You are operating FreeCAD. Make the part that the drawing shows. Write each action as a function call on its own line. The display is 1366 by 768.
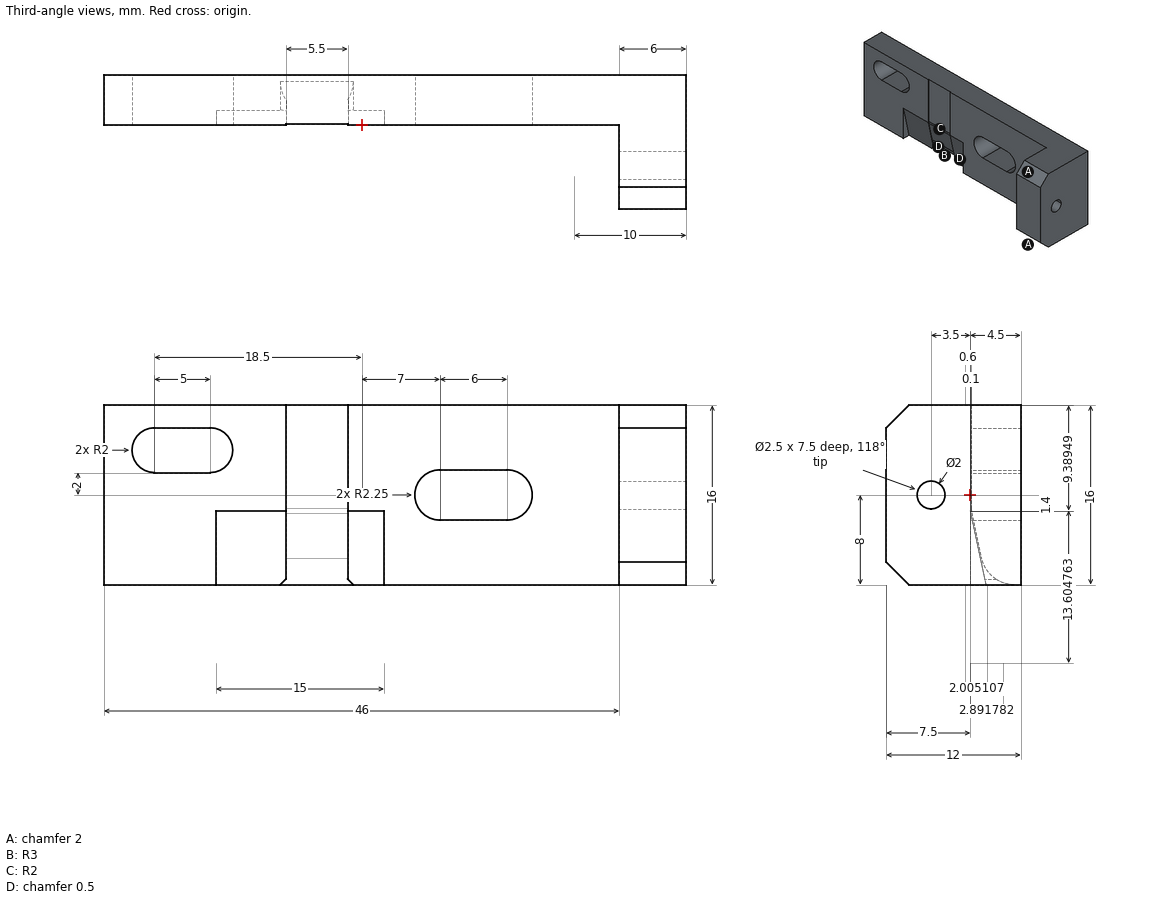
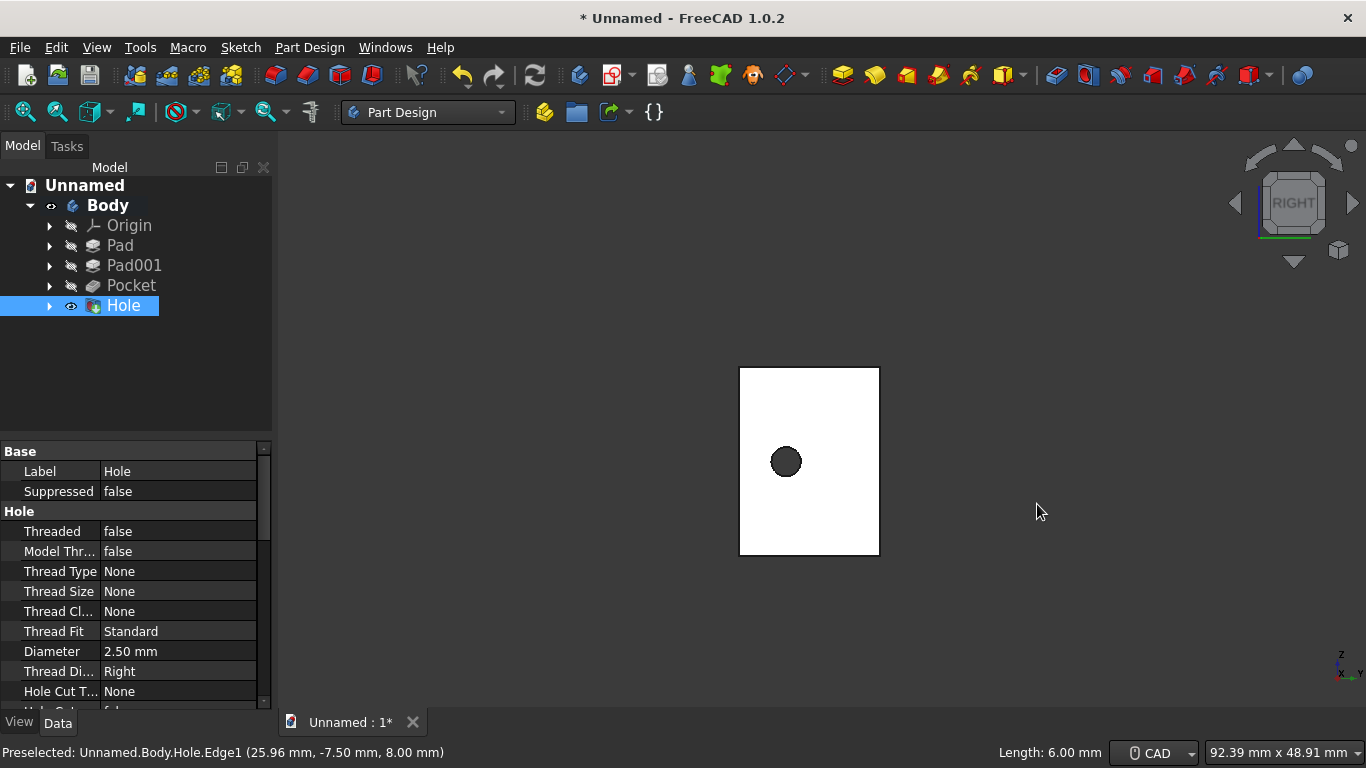
key(v)
key(f)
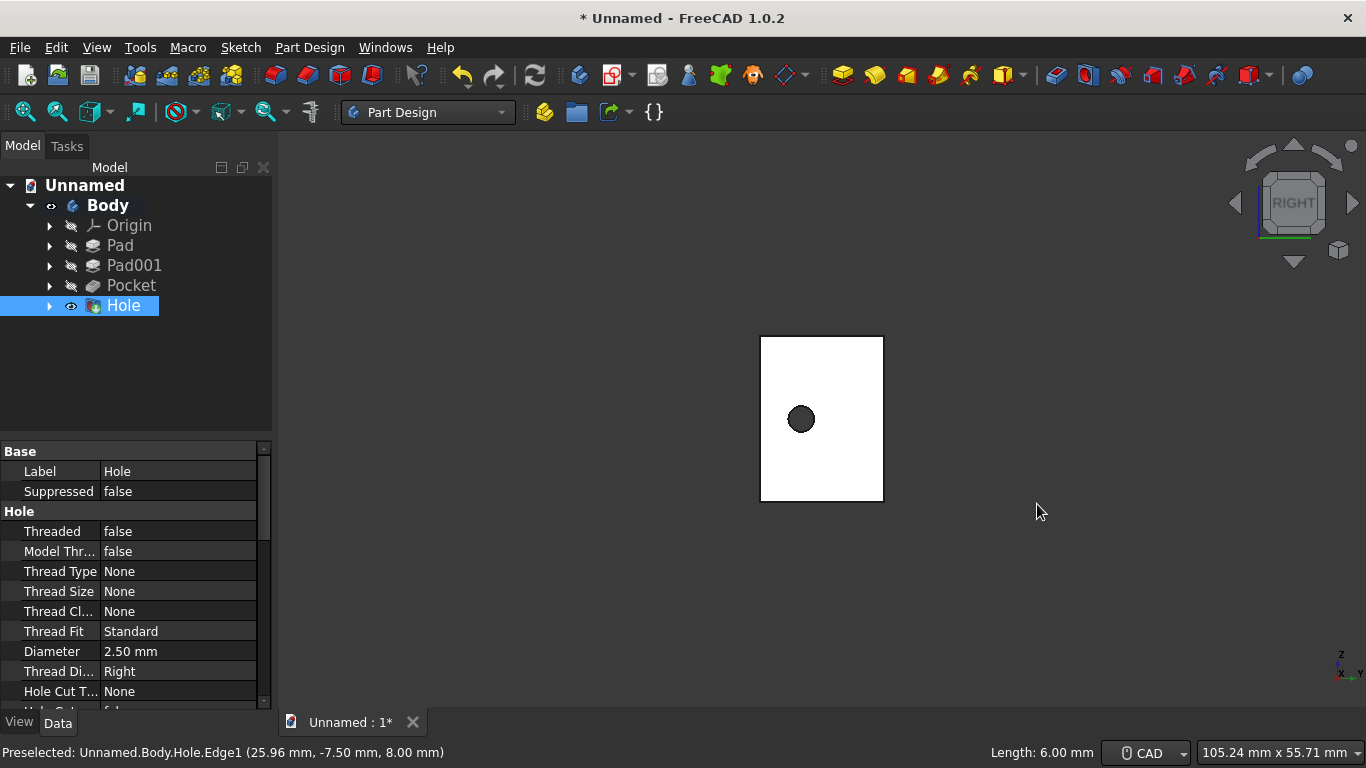
key(5)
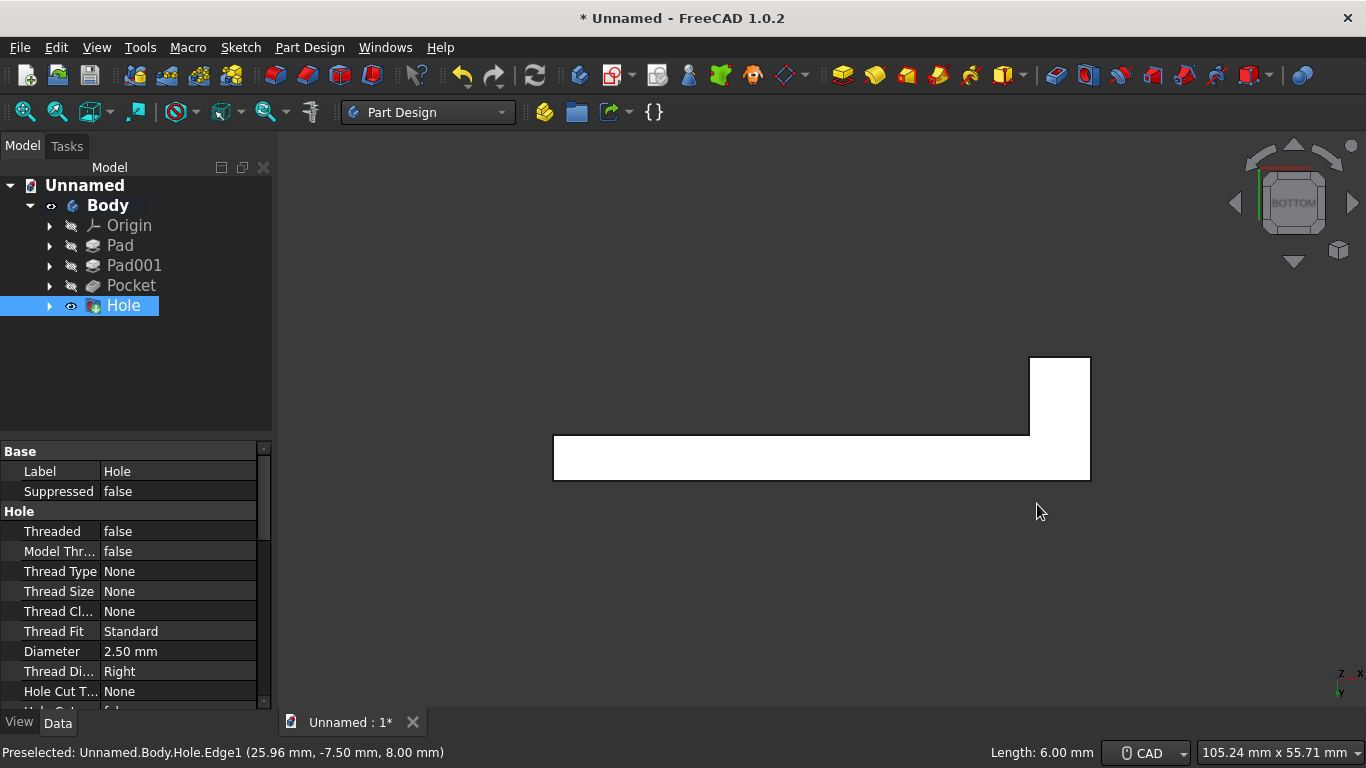
click(1060, 356, ctrl)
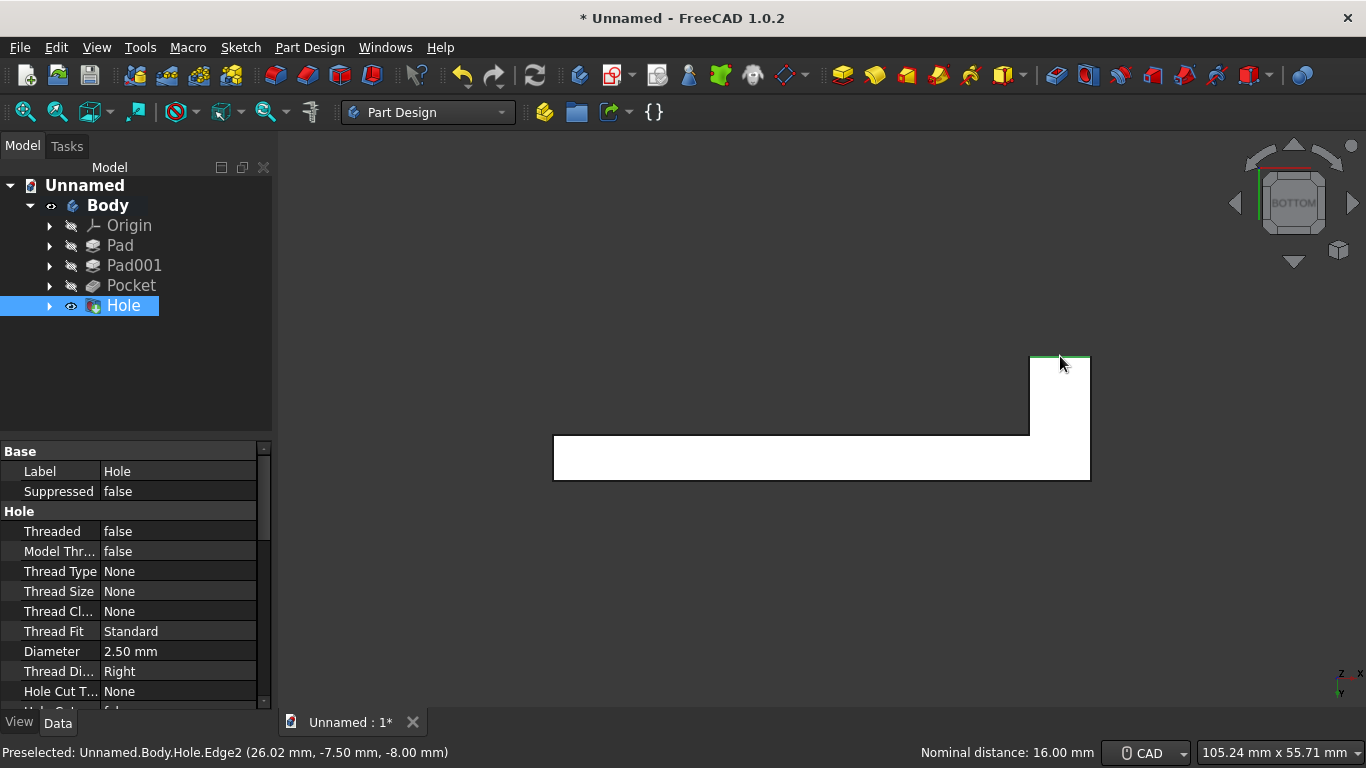
click(308, 76)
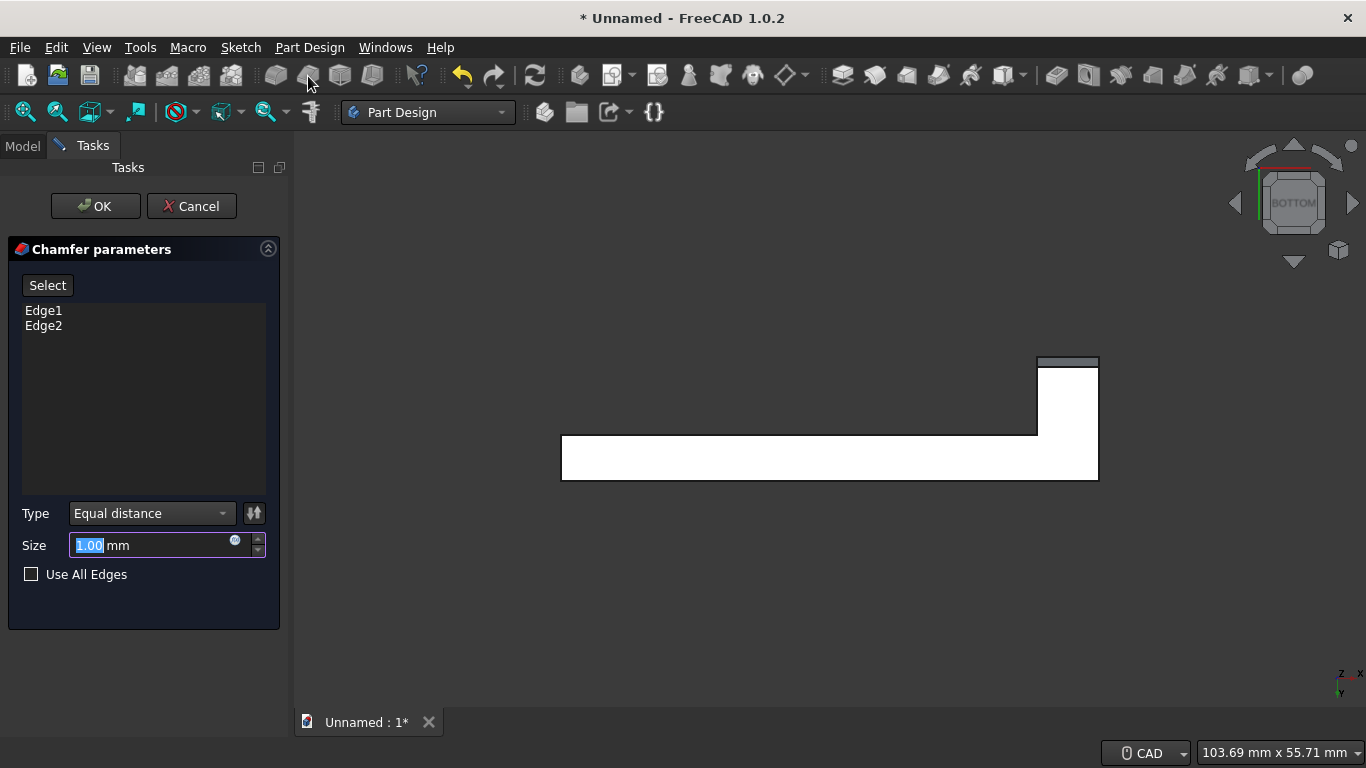
text(2)
key(Tab)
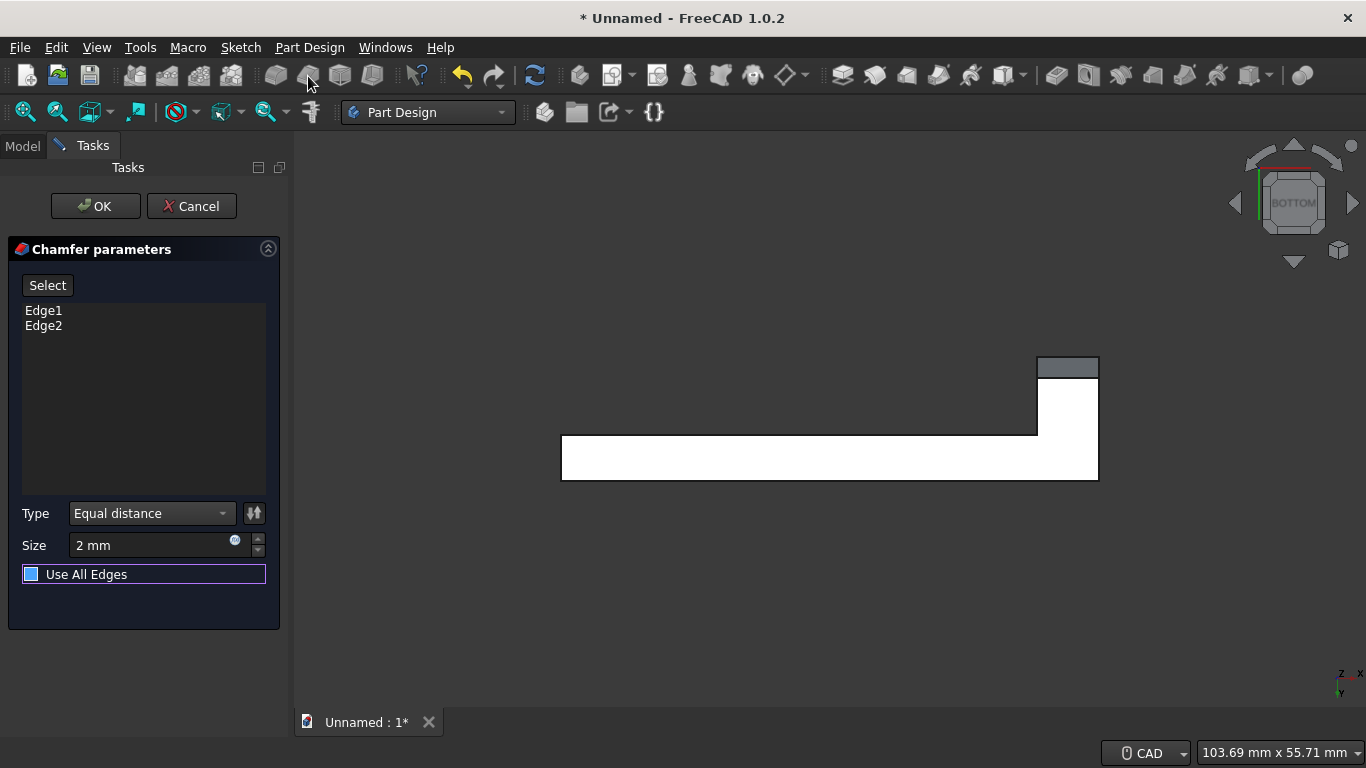
click(96, 206)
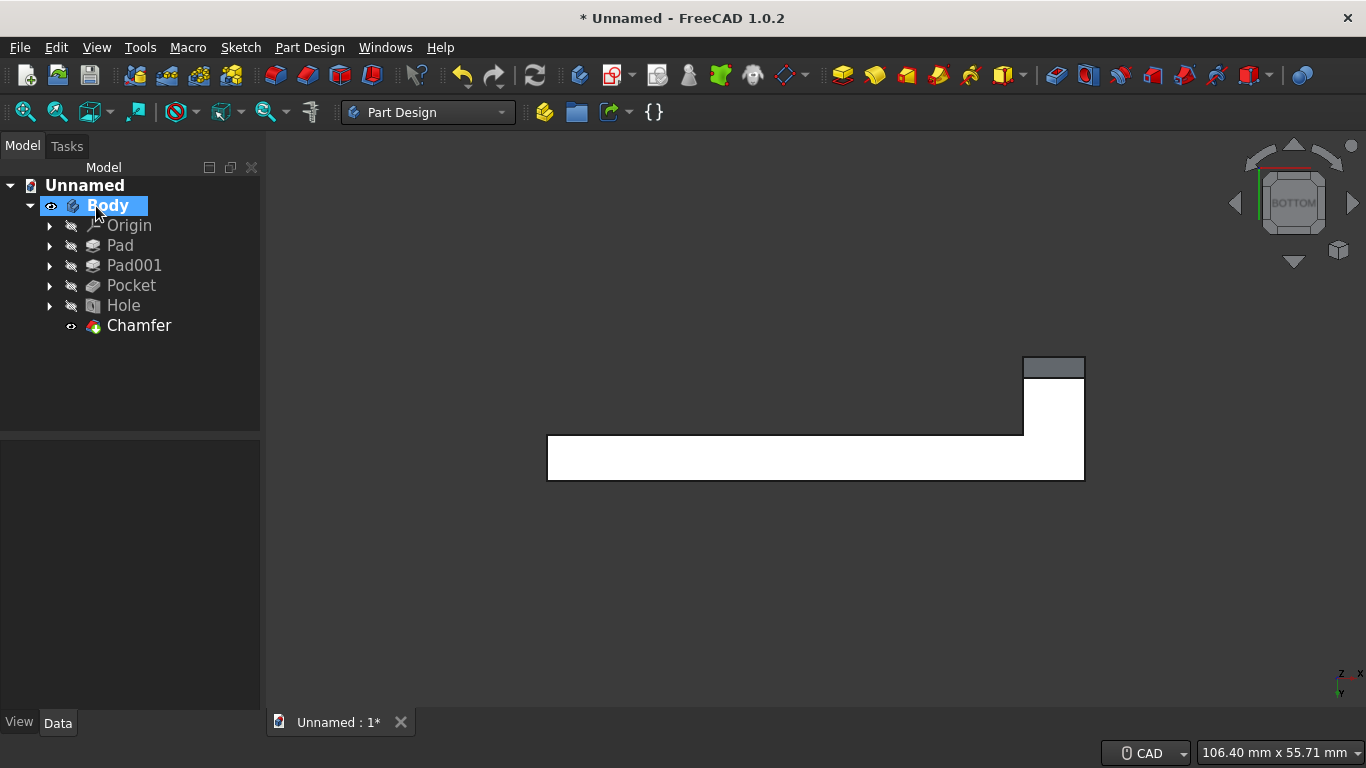
click(50, 226)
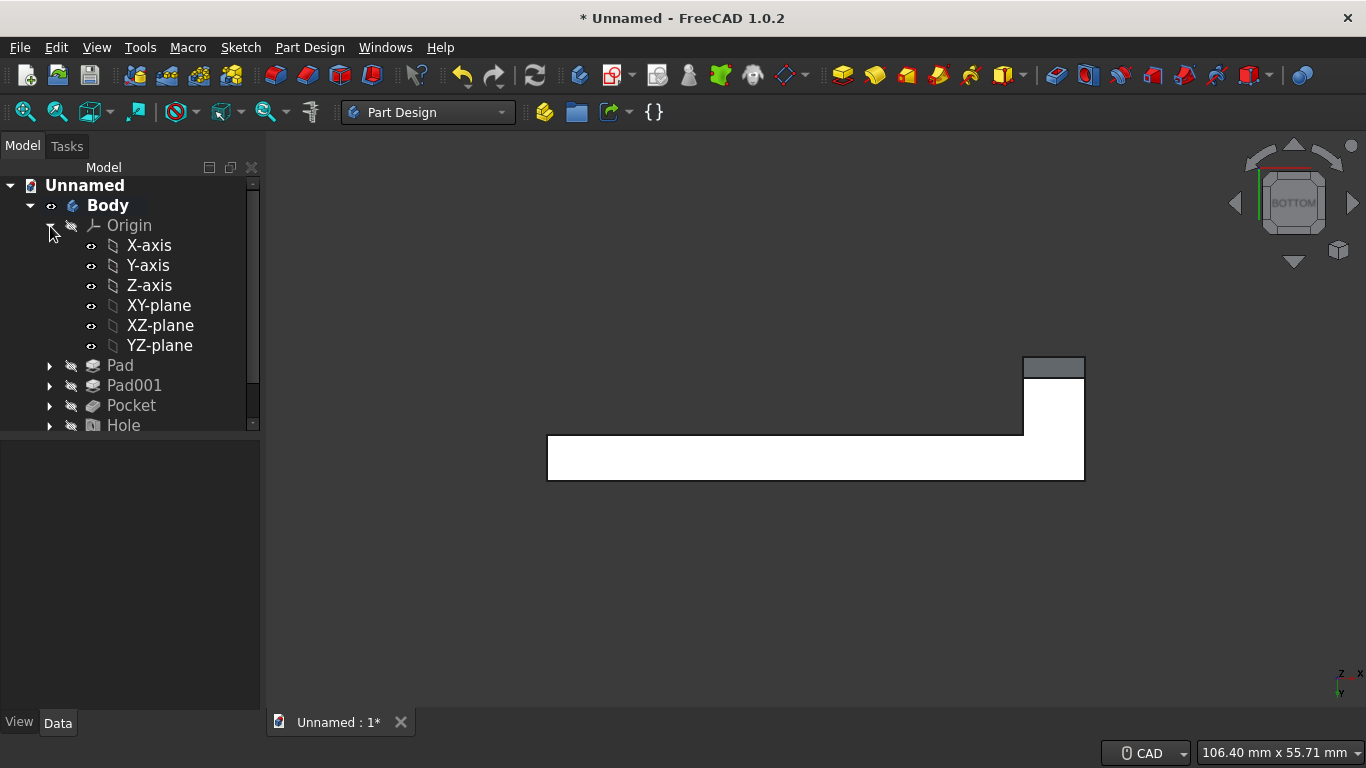
click(136, 346)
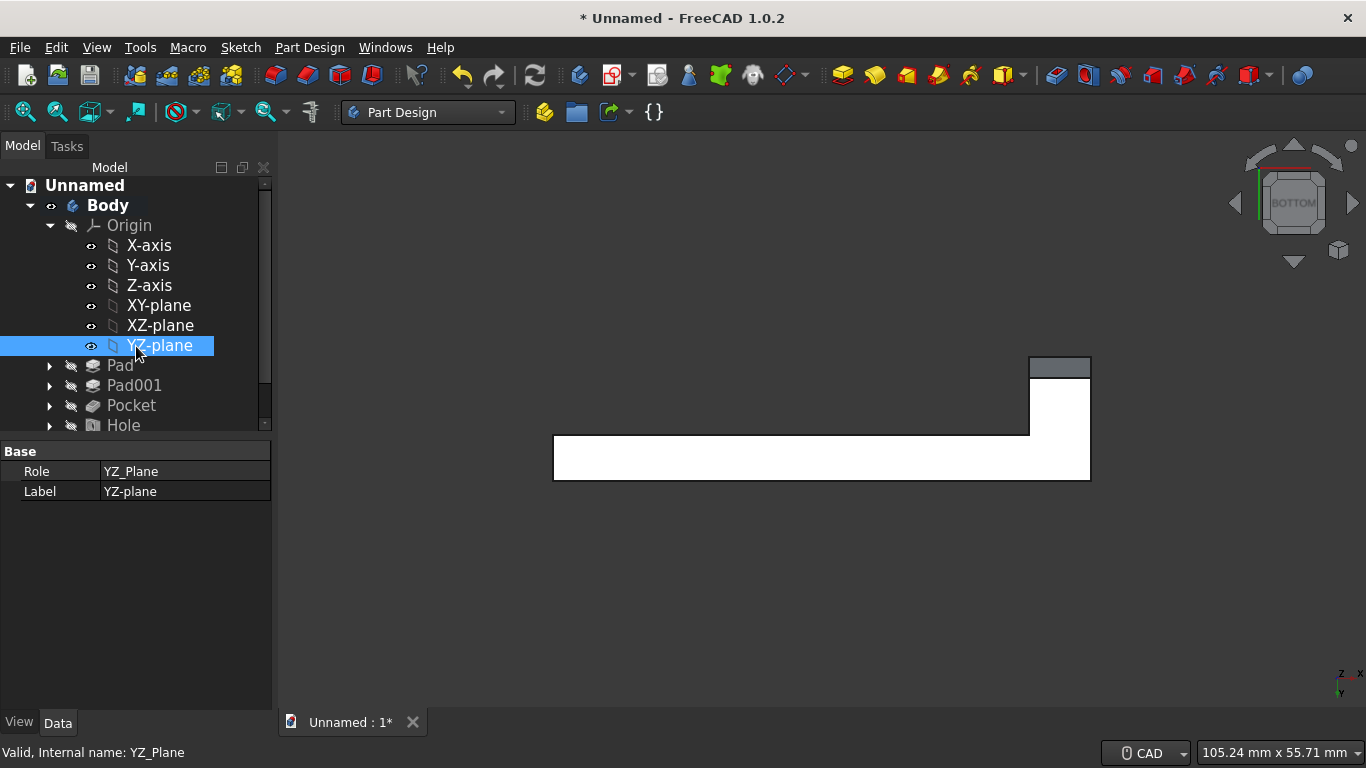
click(786, 76)